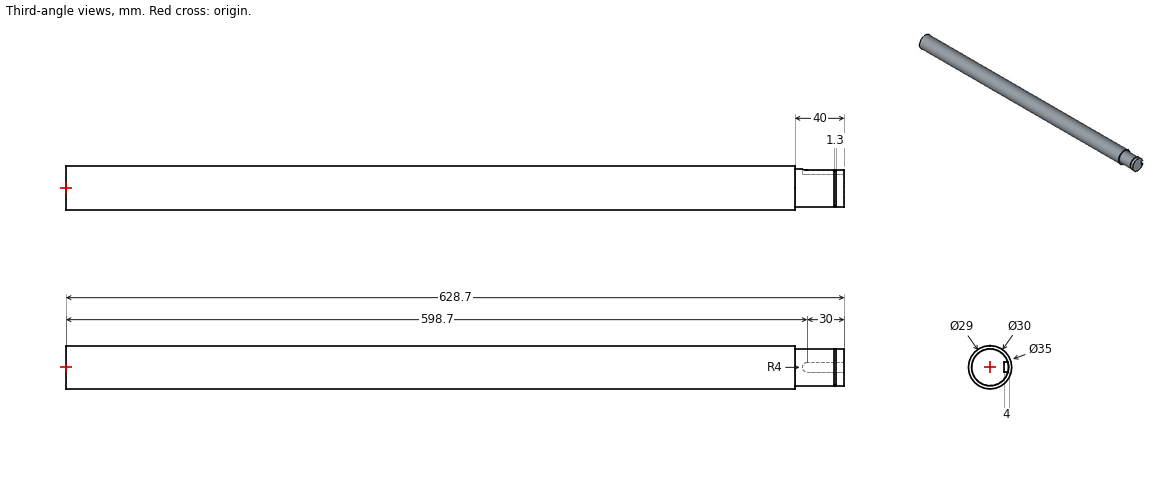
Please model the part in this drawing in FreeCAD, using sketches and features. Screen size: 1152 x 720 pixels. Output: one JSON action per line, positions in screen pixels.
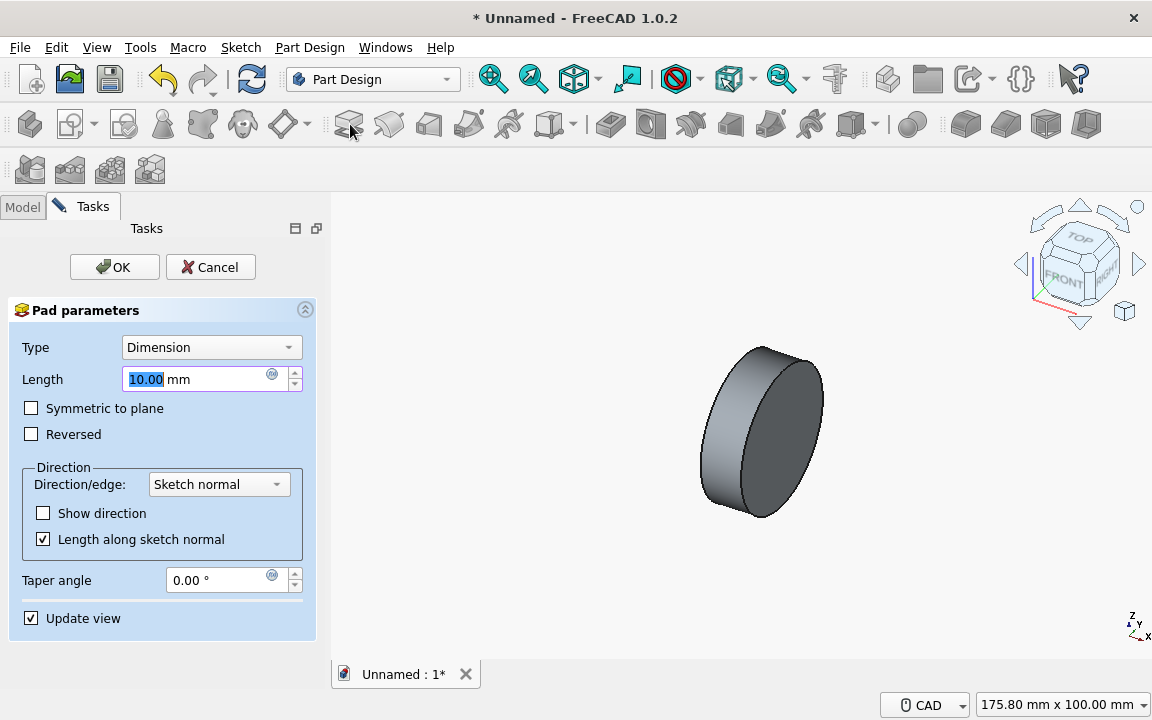
{"action": "type", "text": "628.7"}
{"action": "key", "text": "Tab"}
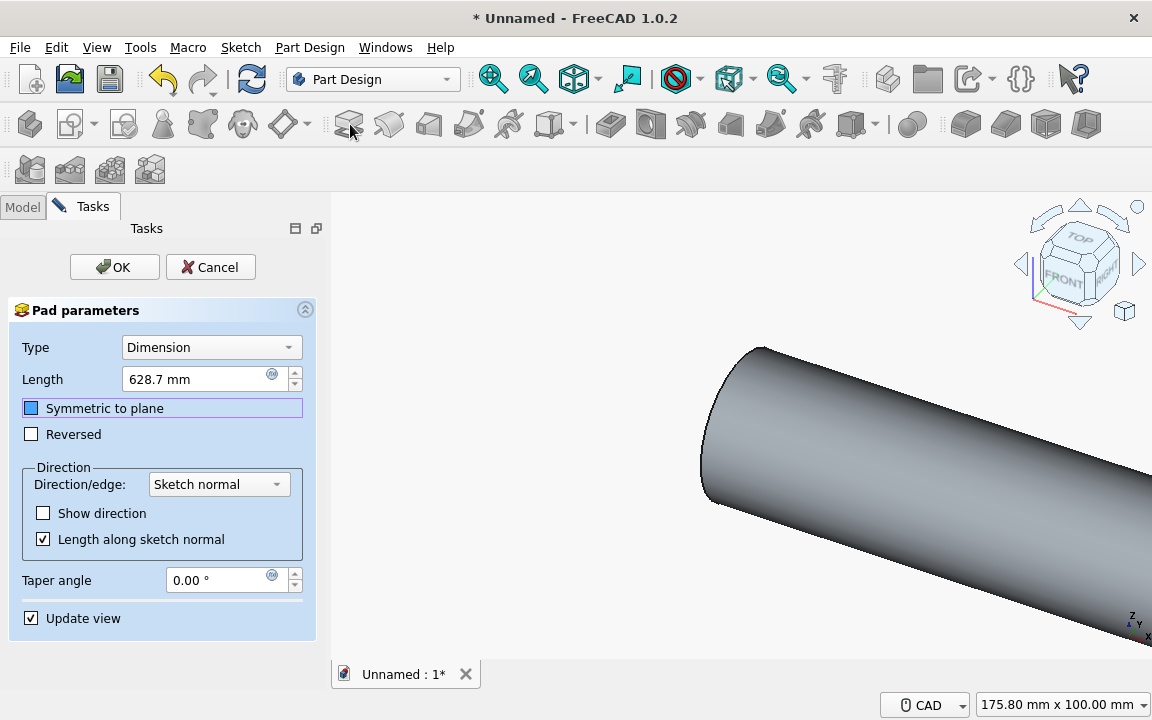
{"action": "left_click", "coordinate": [115, 267]}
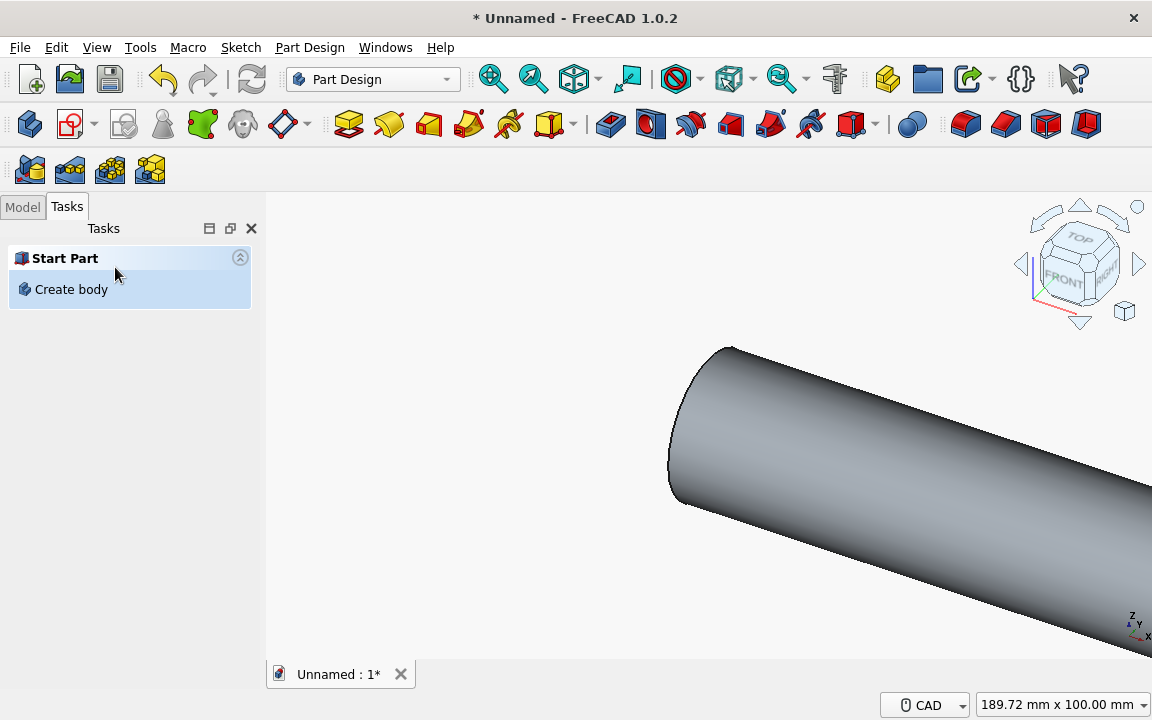
{"action": "left_click", "coordinate": [494, 80]}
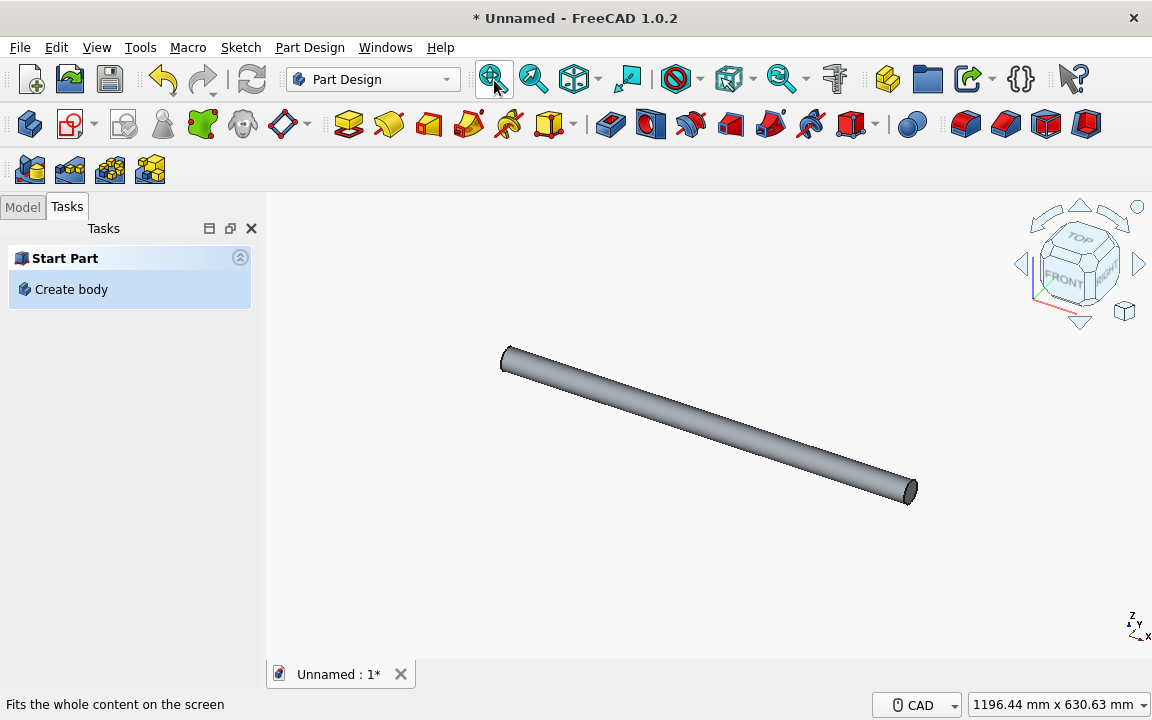
{"action": "left_click", "coordinate": [23, 206]}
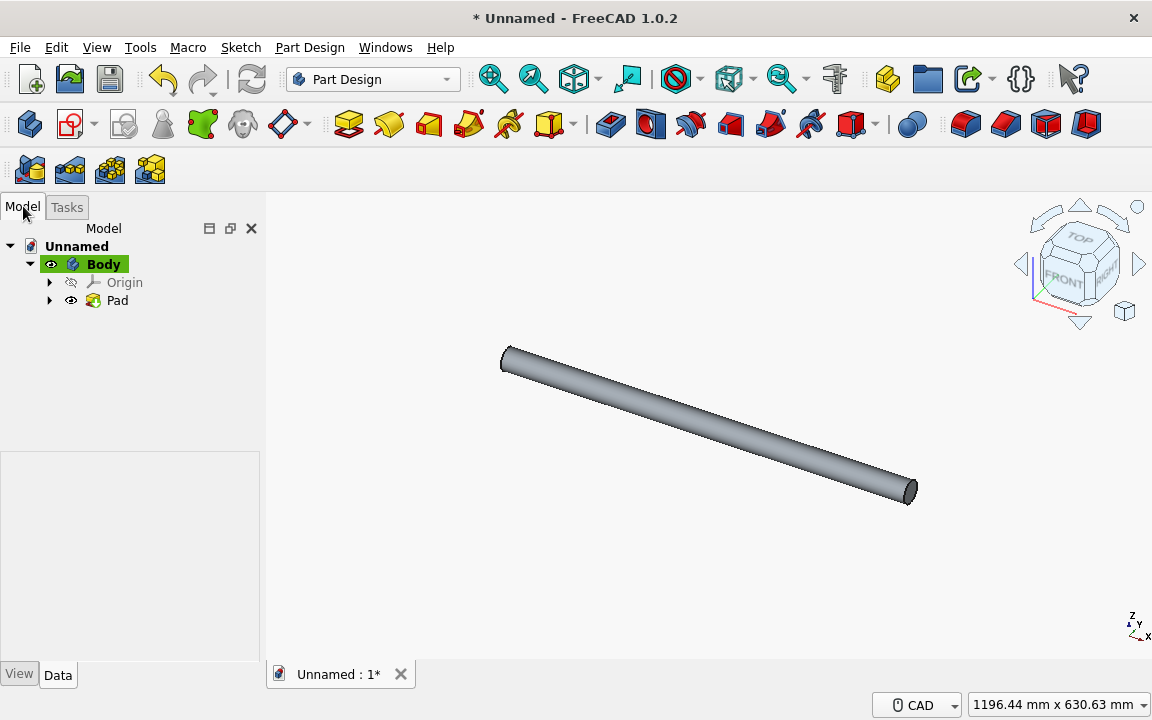
{"action": "left_click", "coordinate": [50, 282]}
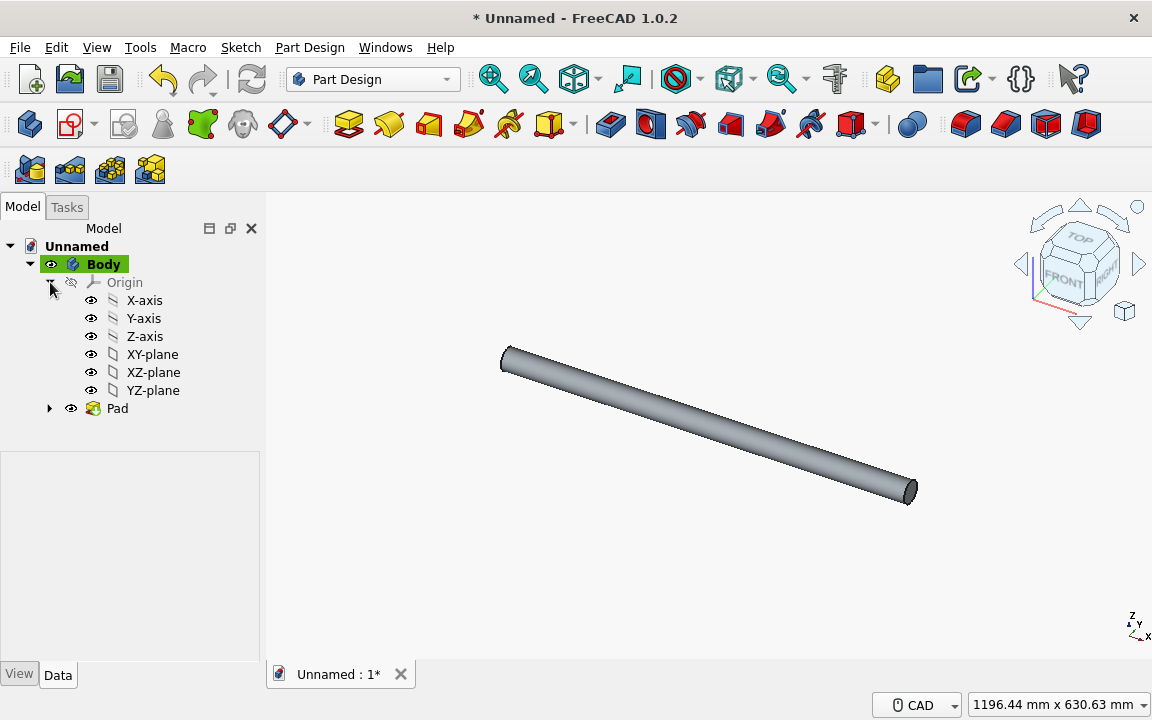
{"action": "left_click", "coordinate": [136, 390]}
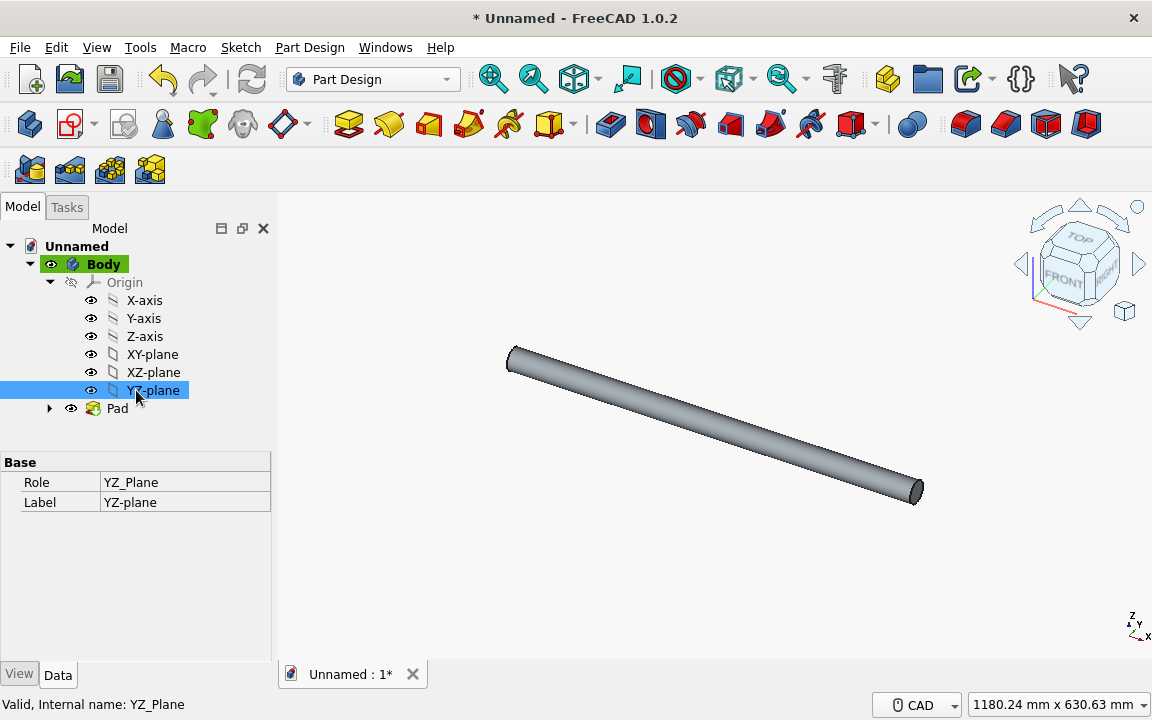
{"action": "left_click", "coordinate": [284, 124]}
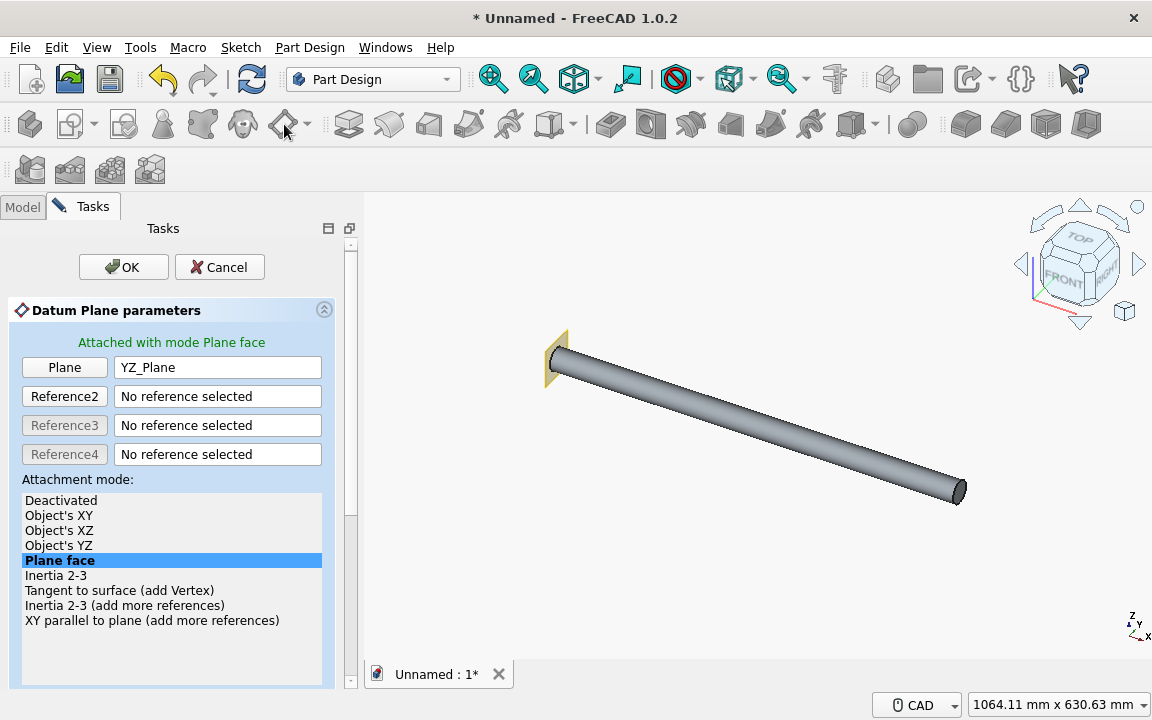
{"action": "scroll", "coordinate": [351, 463], "scroll_direction": "down", "scroll_amount": 3}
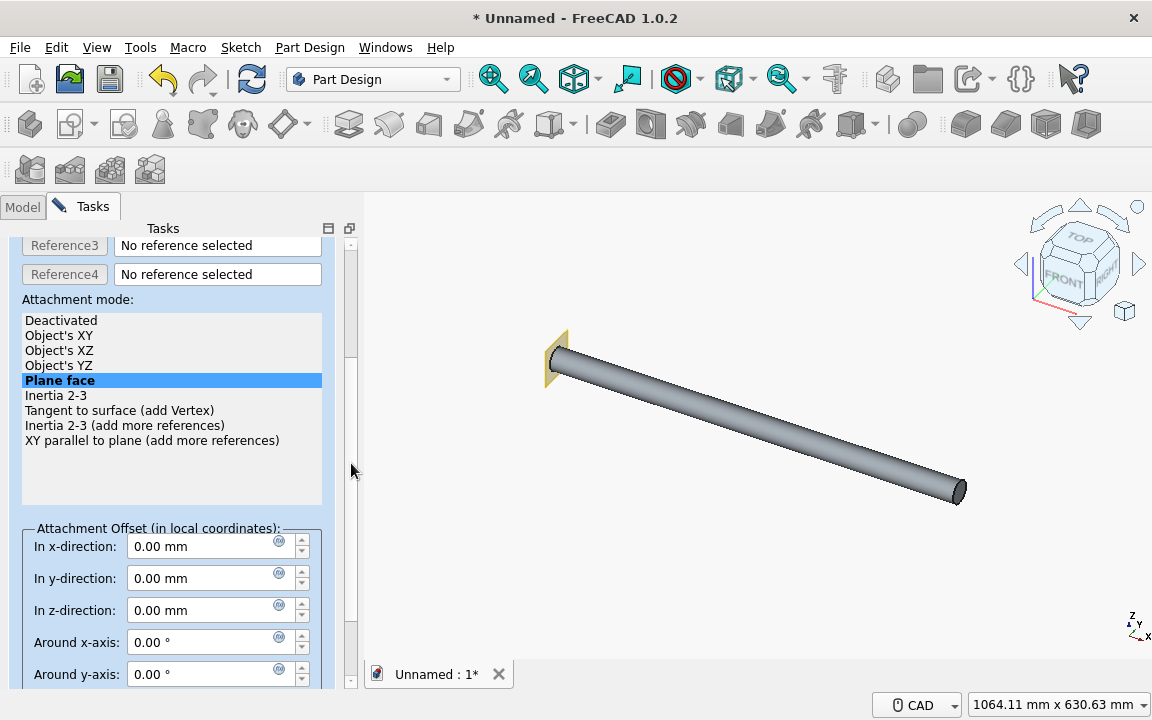
{"action": "triple_click", "coordinate": [210, 610]}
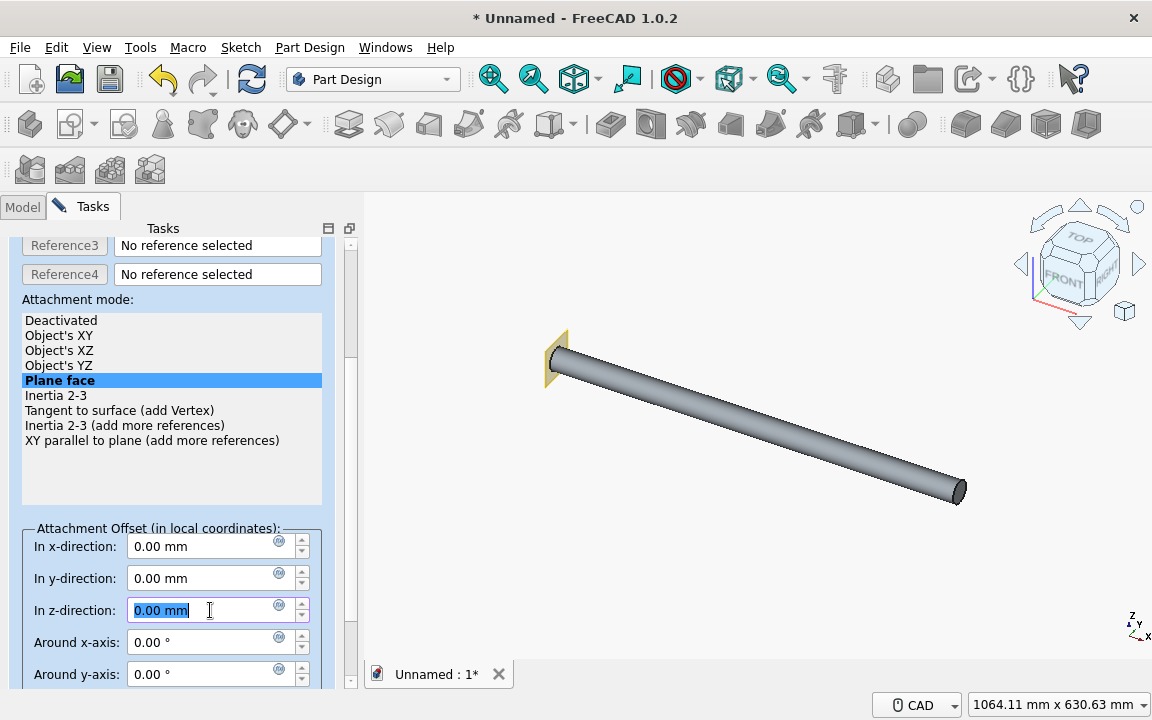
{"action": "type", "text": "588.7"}
{"action": "key", "text": "Tab"}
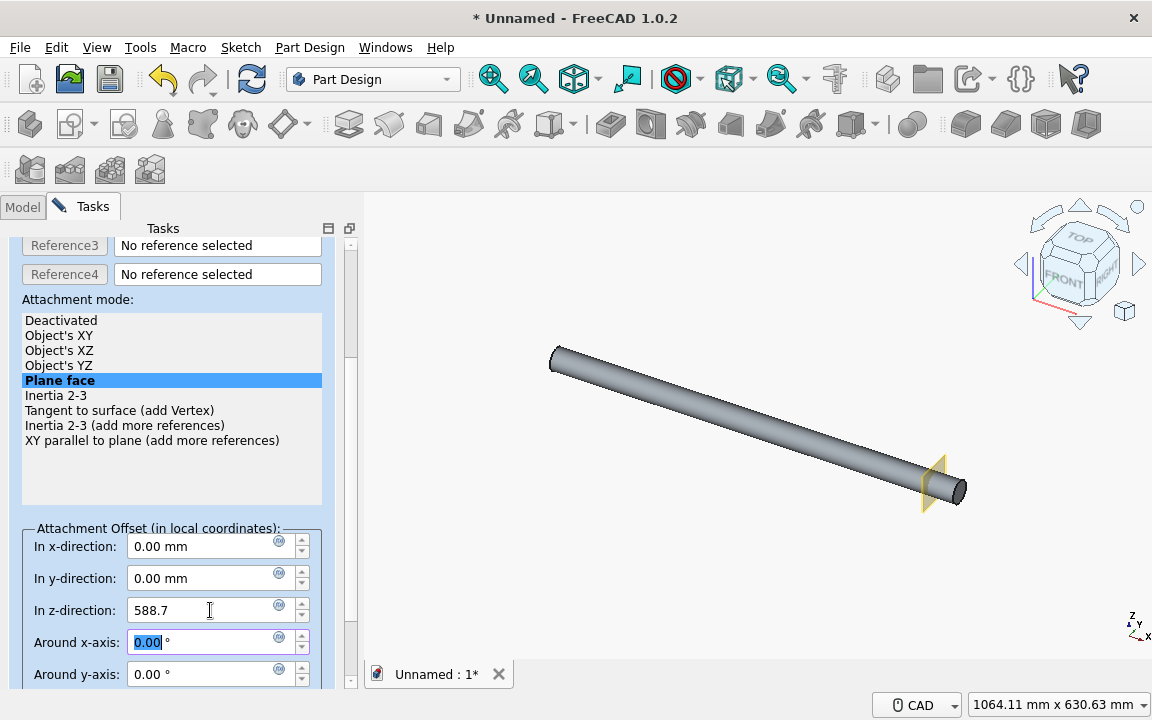
{"action": "scroll", "coordinate": [351, 463], "scroll_direction": "up", "scroll_amount": 4}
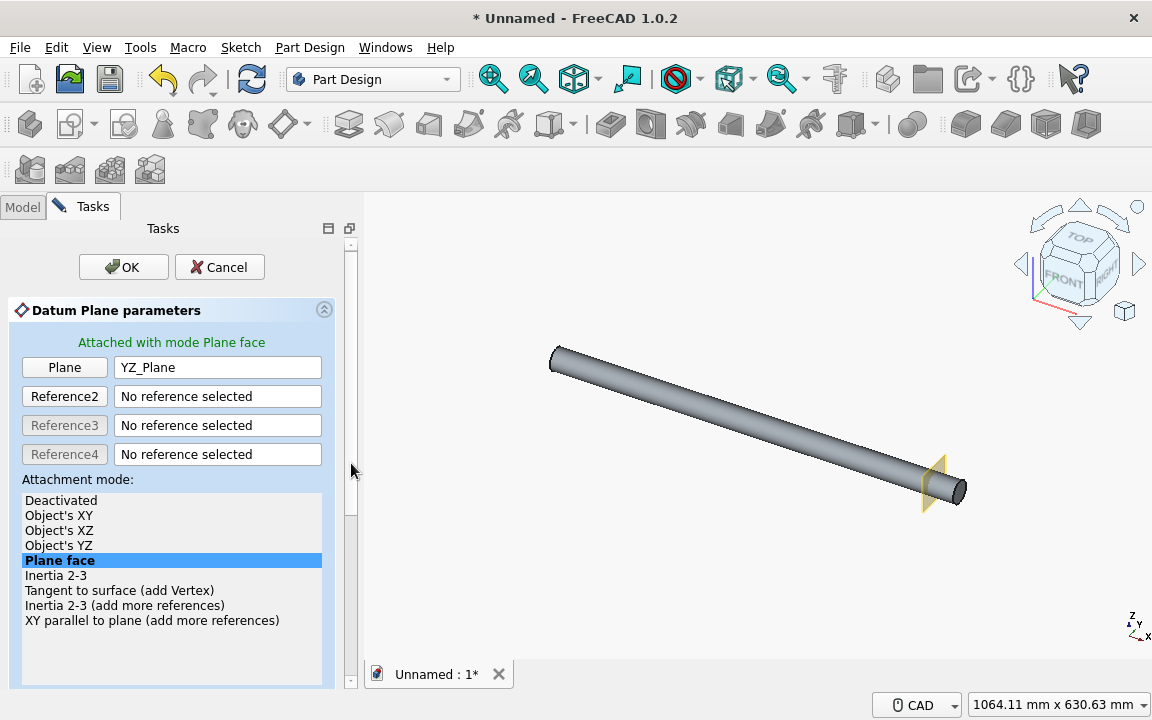
{"action": "left_click", "coordinate": [124, 267]}